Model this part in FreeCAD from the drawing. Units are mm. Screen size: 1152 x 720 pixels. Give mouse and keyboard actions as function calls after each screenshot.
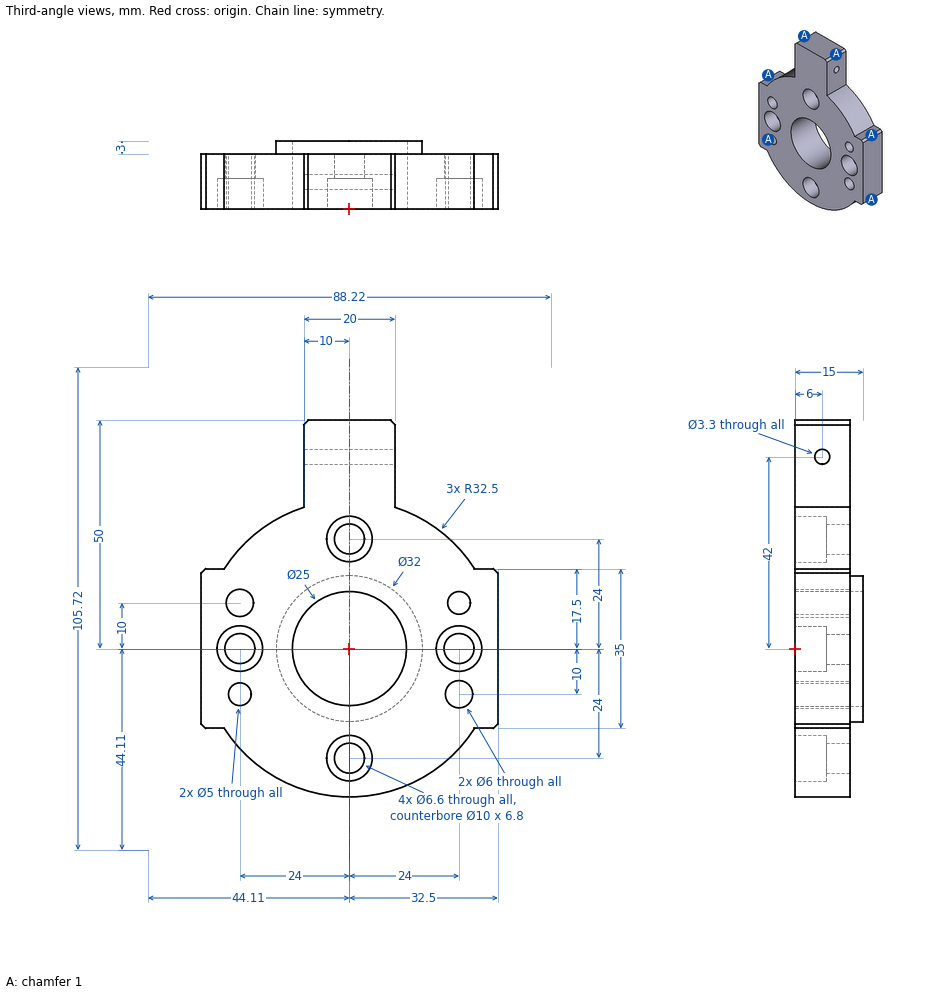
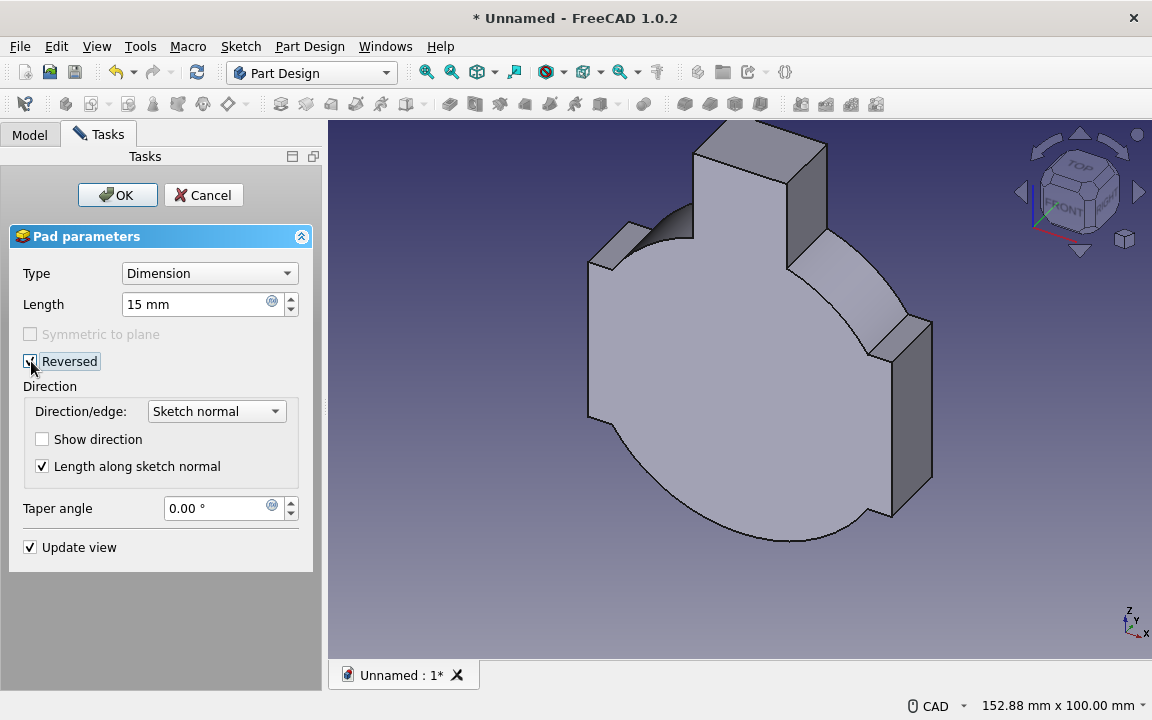
click(118, 195)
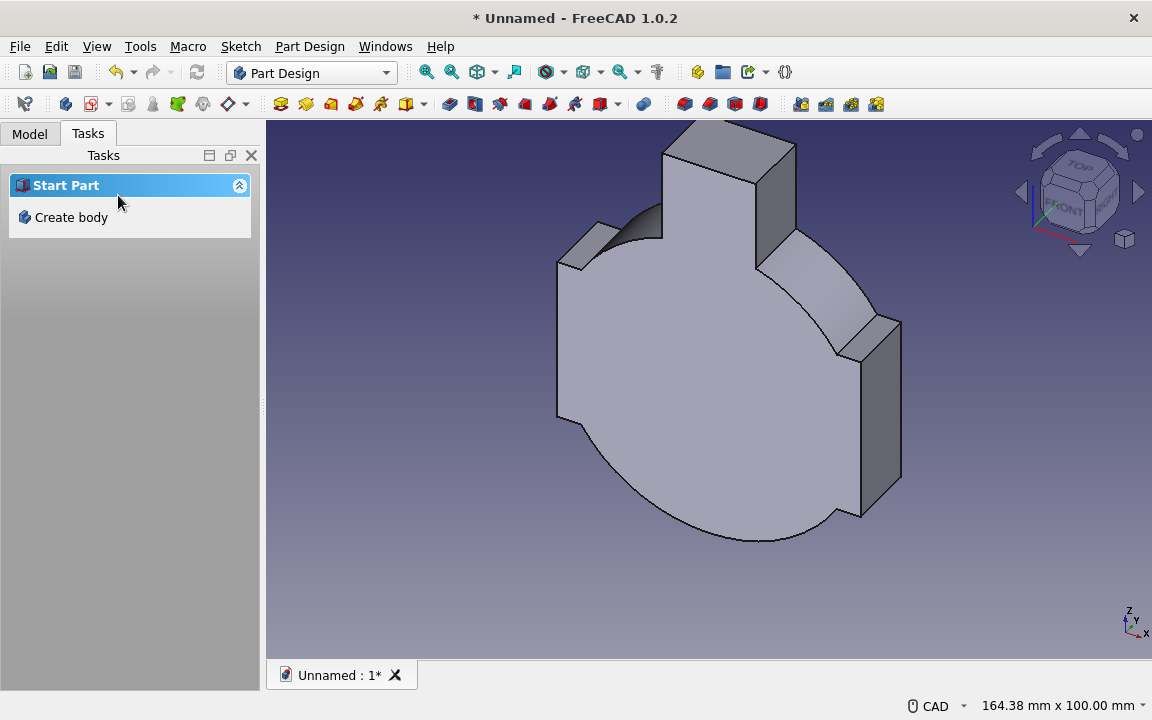
click(427, 72)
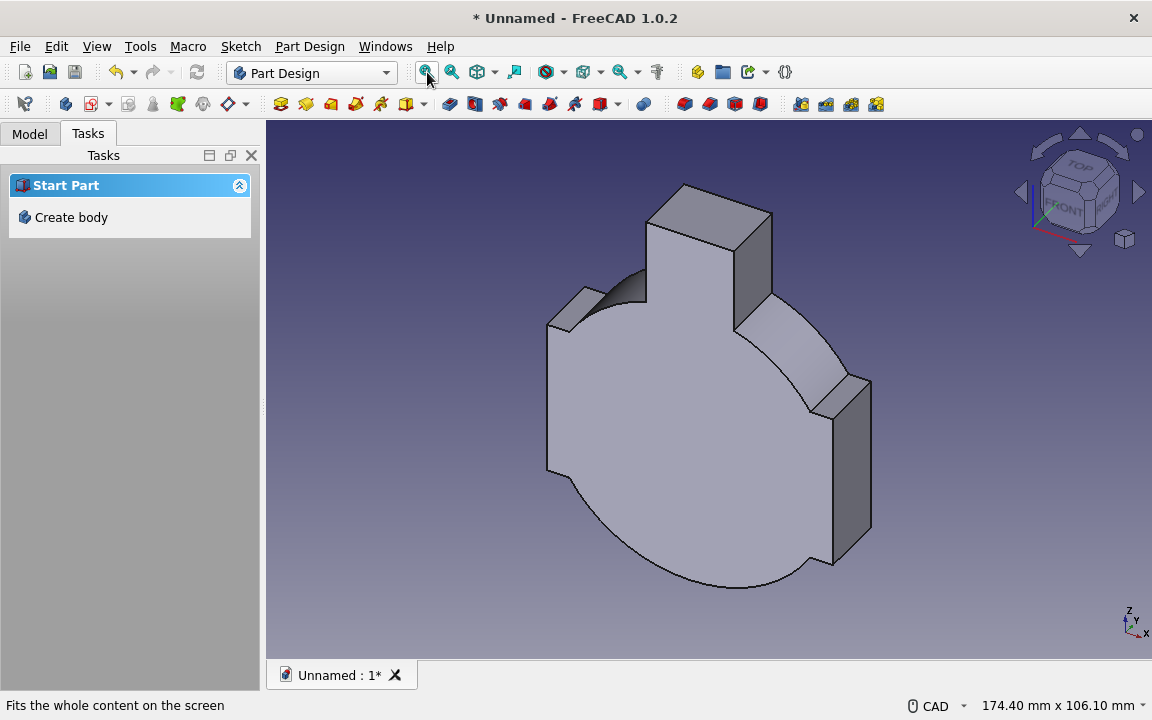
key(4)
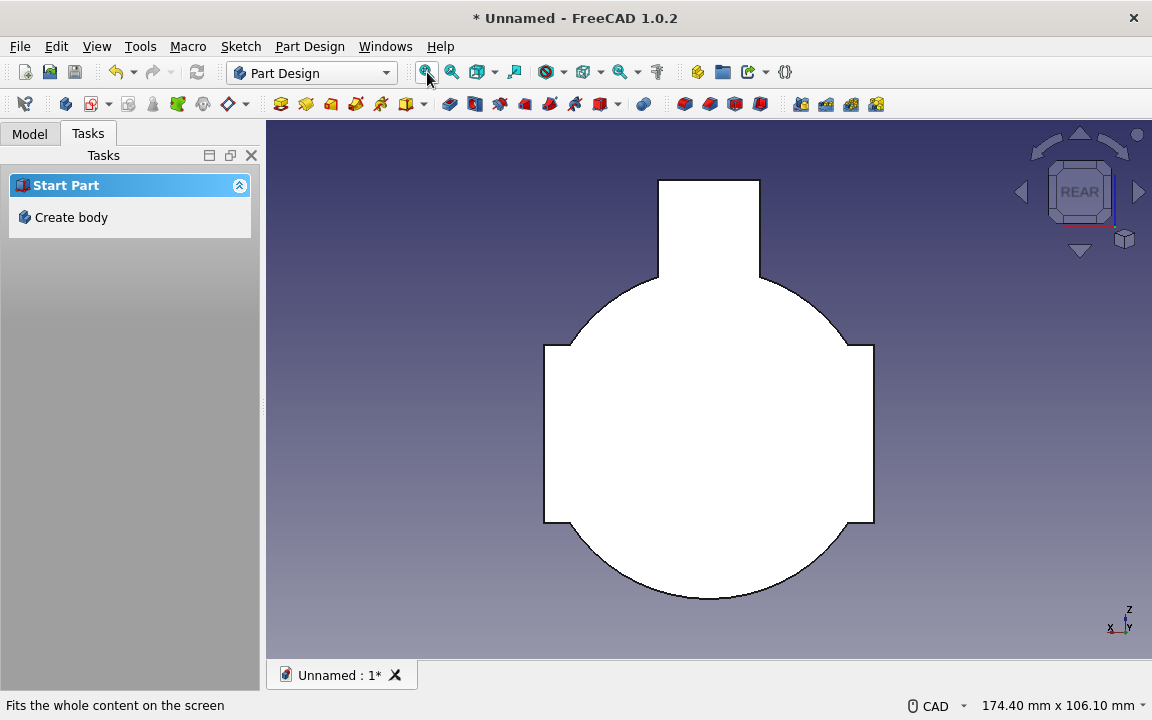
click(709, 448)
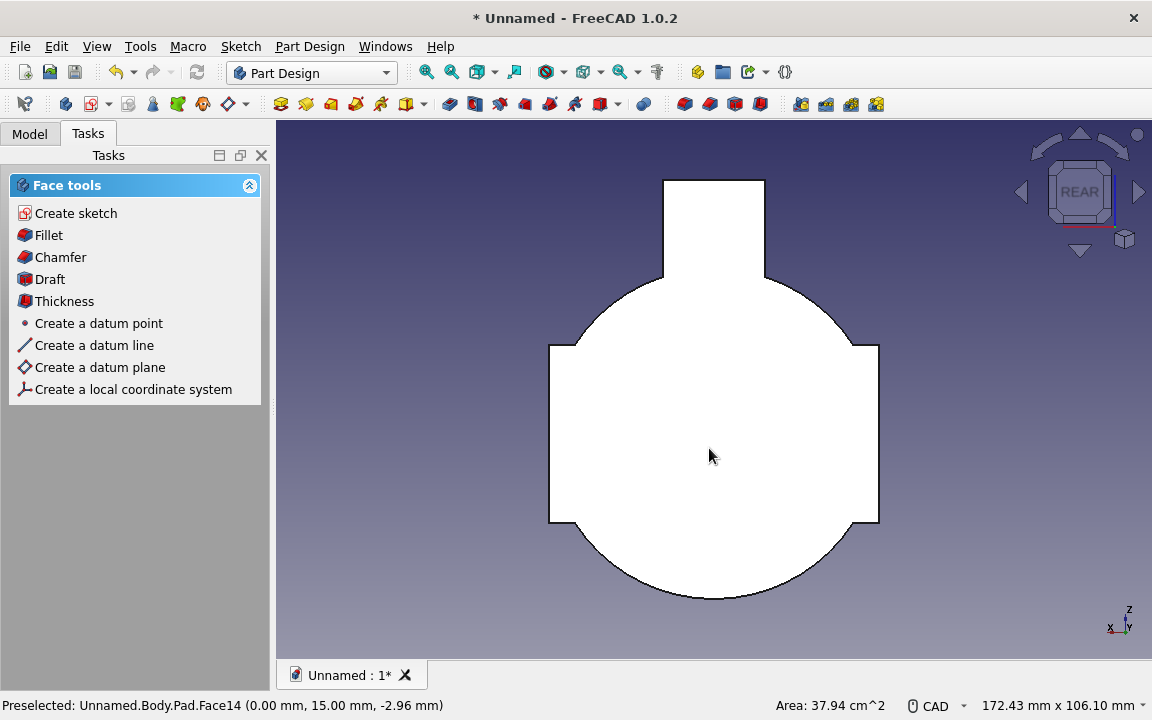
click(90, 104)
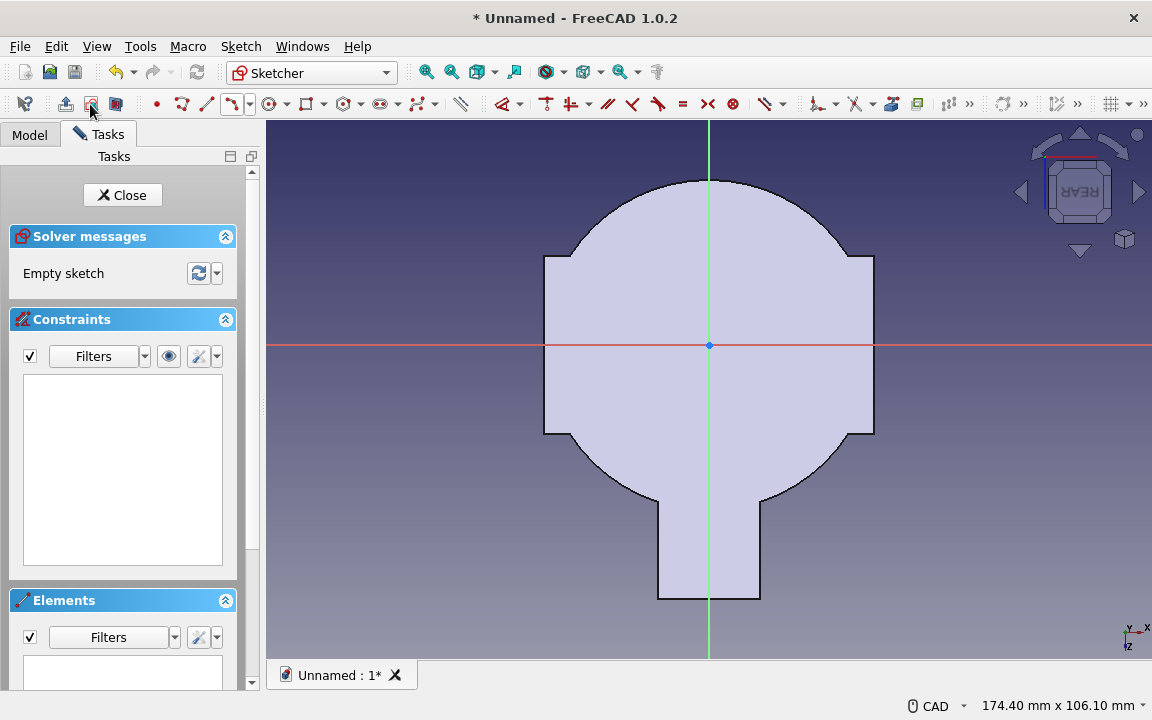
scroll(501, 390, down, 2)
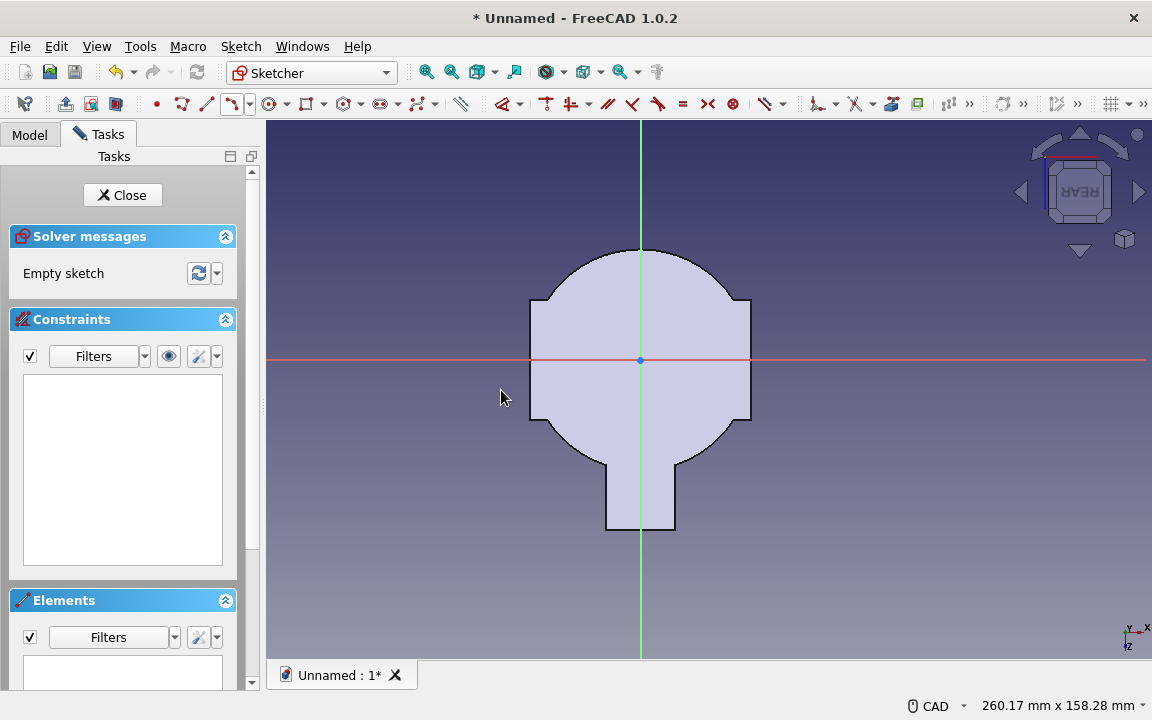
click(306, 104)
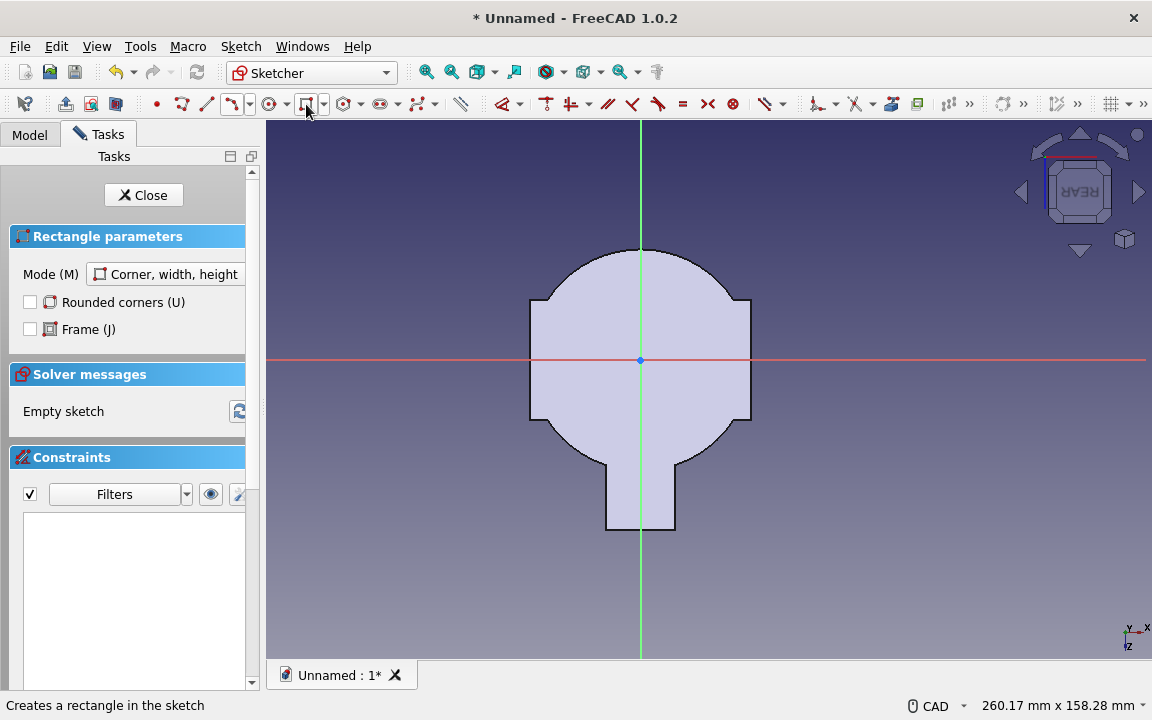
click(490, 210)
click(791, 570)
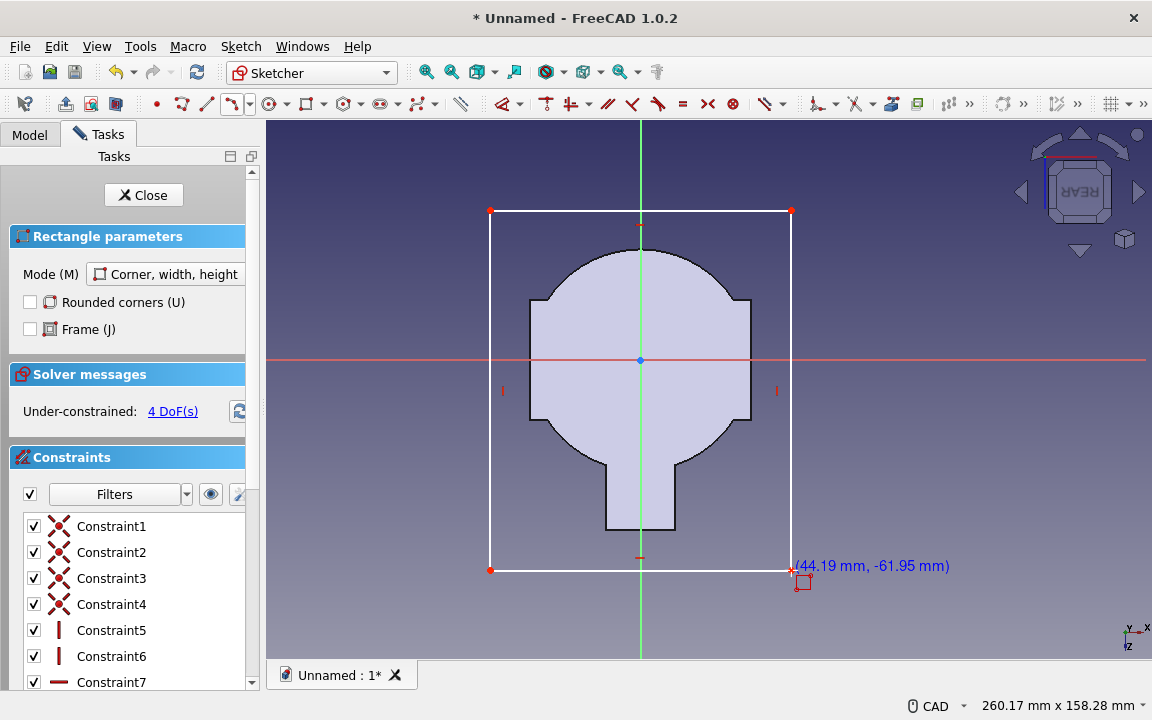
click(268, 104)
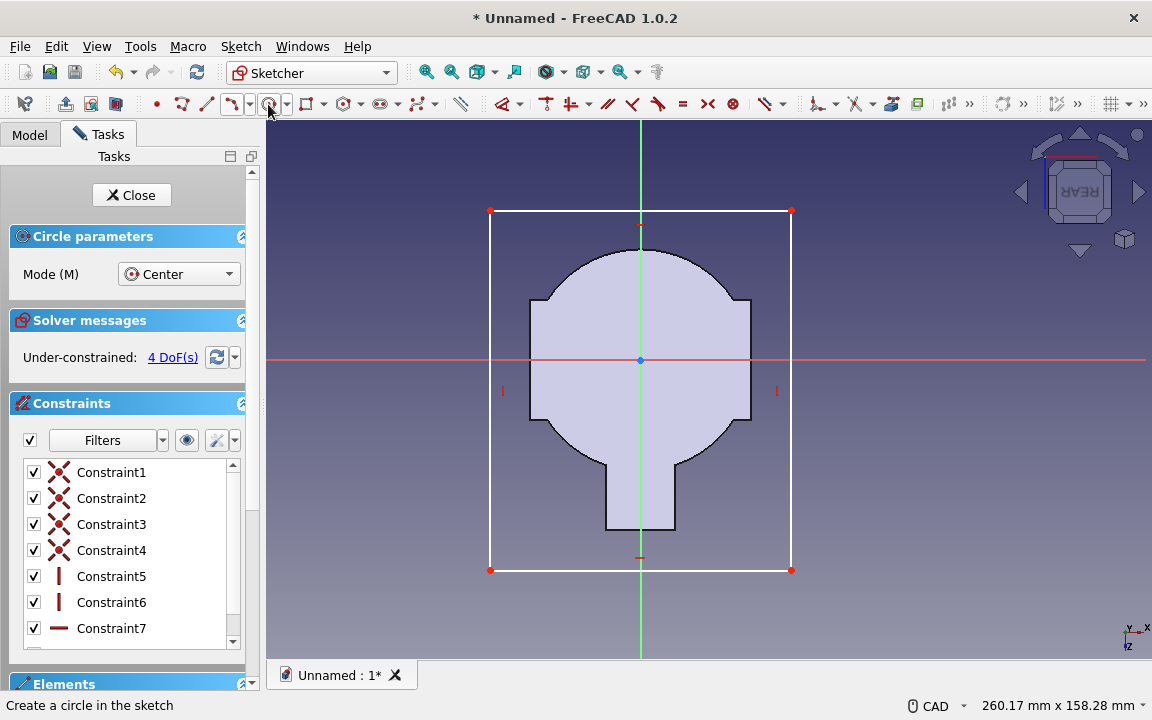
click(641, 360)
click(679, 322)
key(Escape)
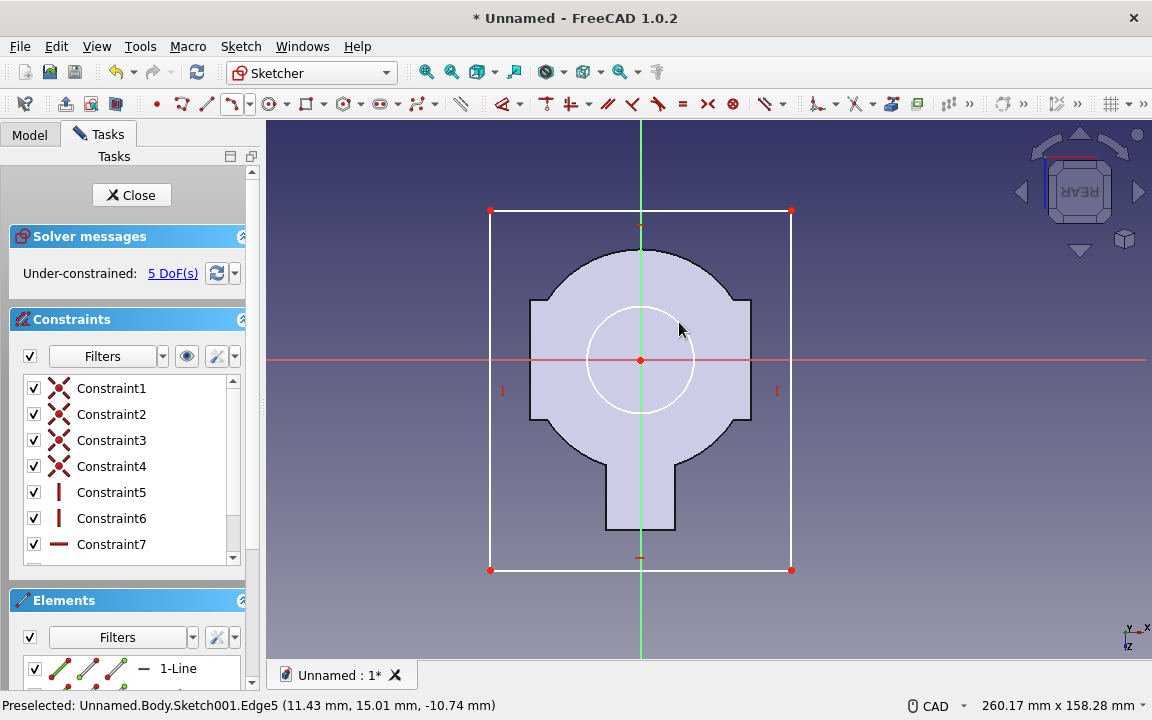
click(502, 104)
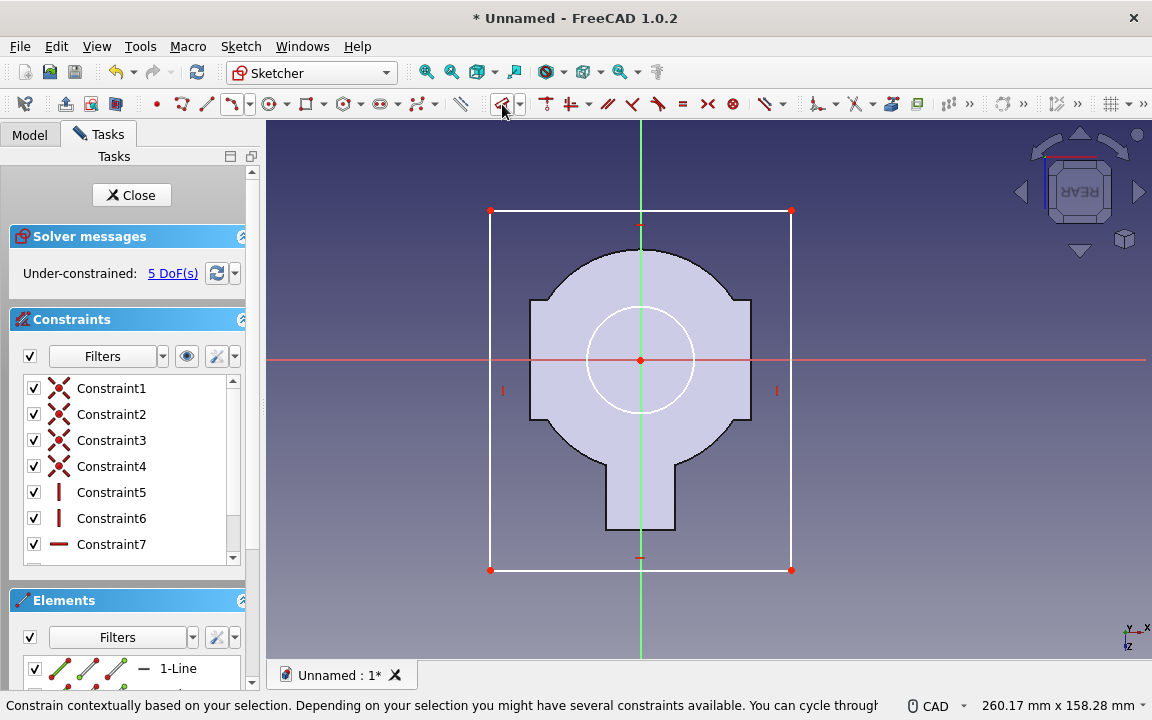
click(678, 322)
click(700, 299)